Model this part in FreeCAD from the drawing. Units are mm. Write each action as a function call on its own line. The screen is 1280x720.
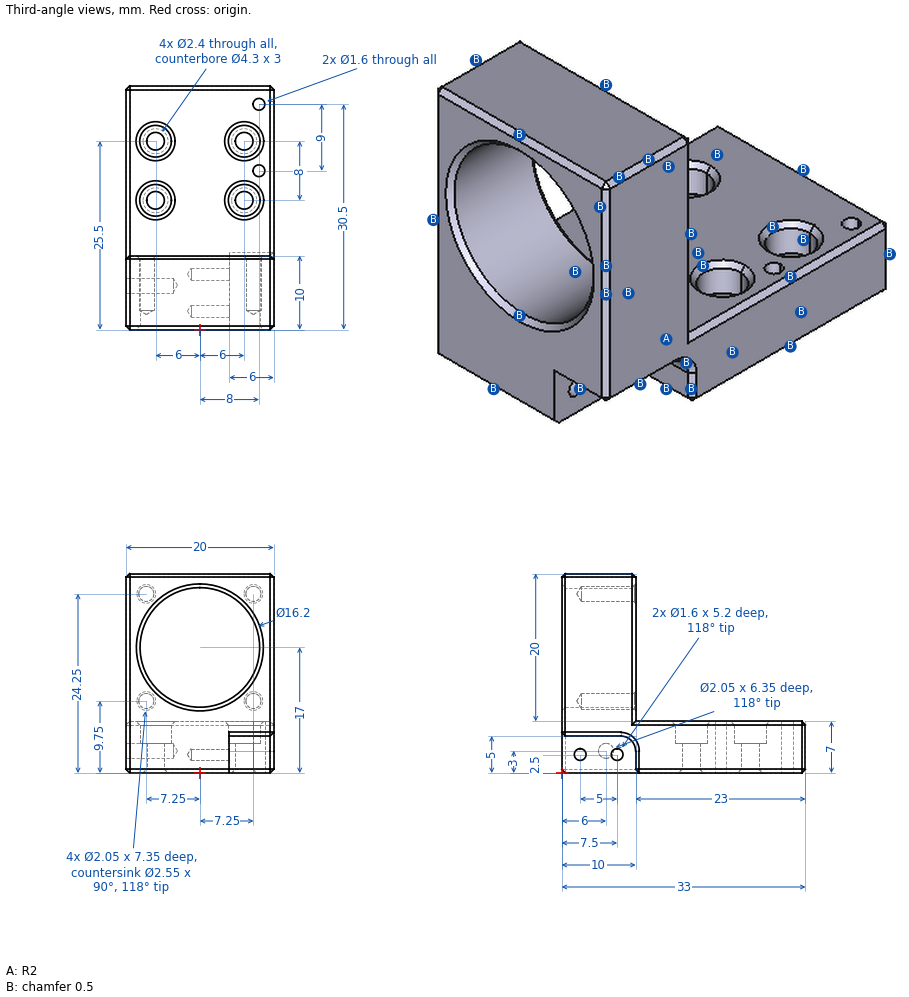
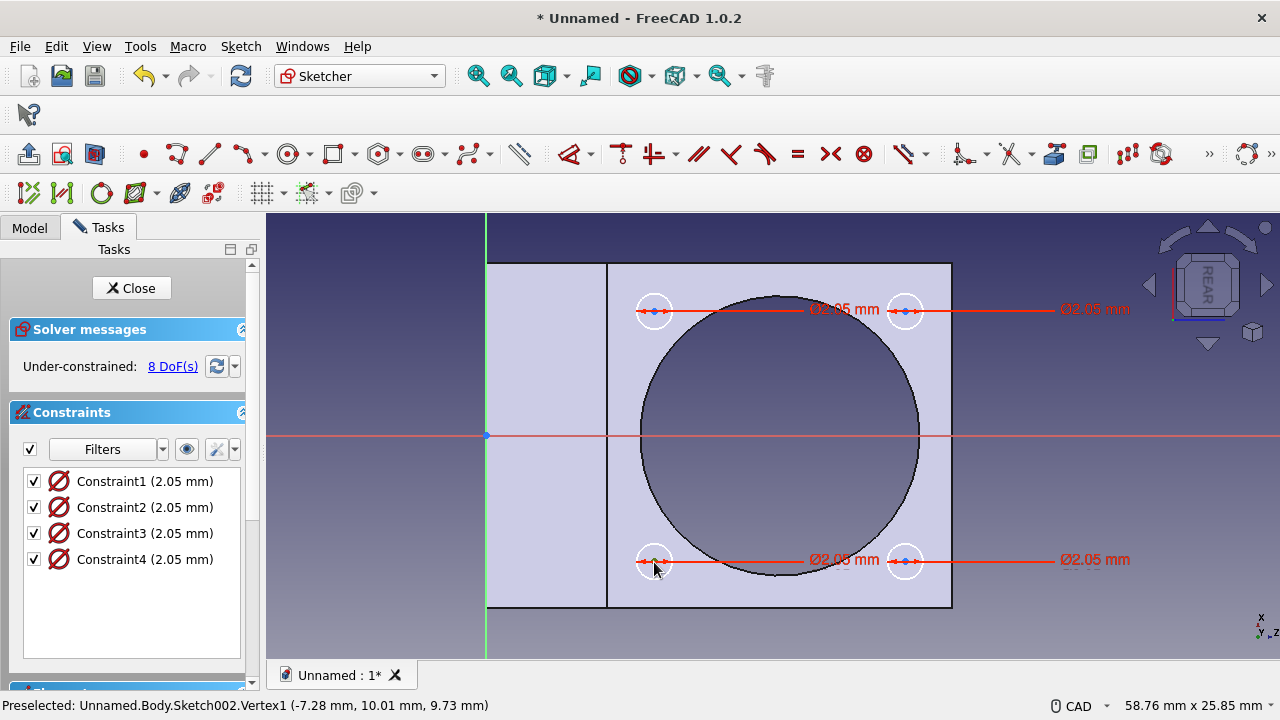
click(905, 562)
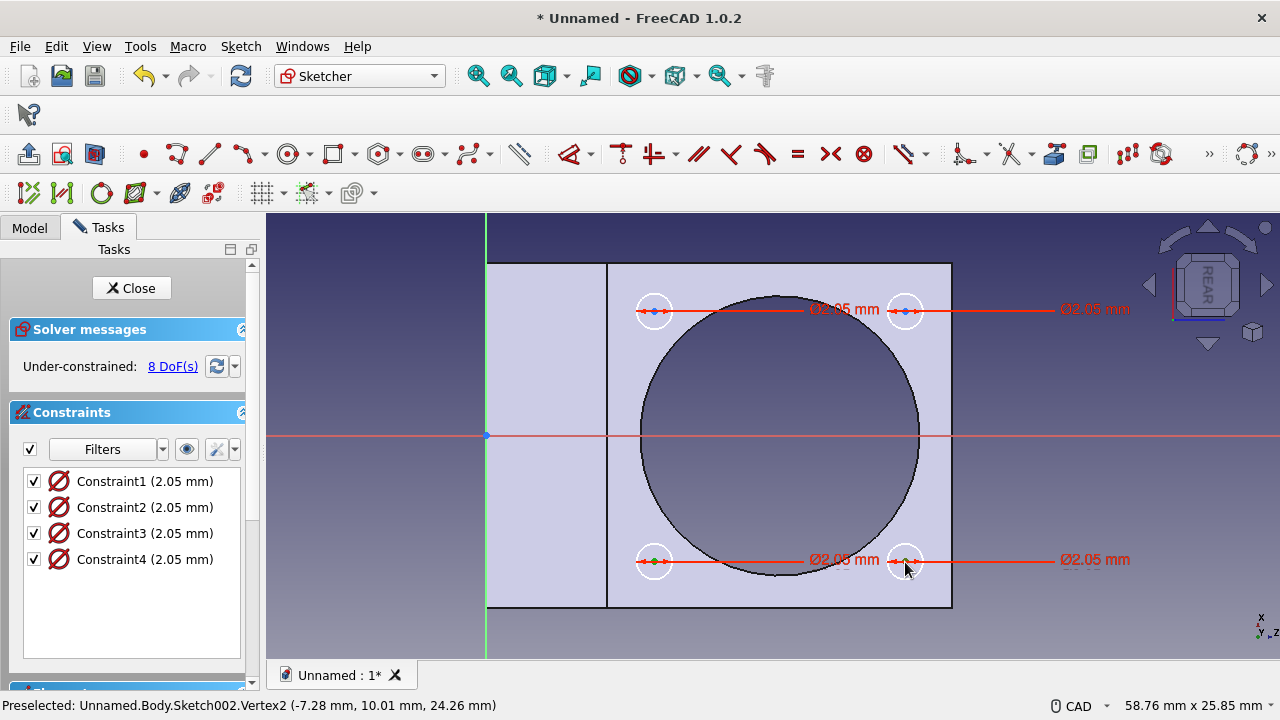
key(h)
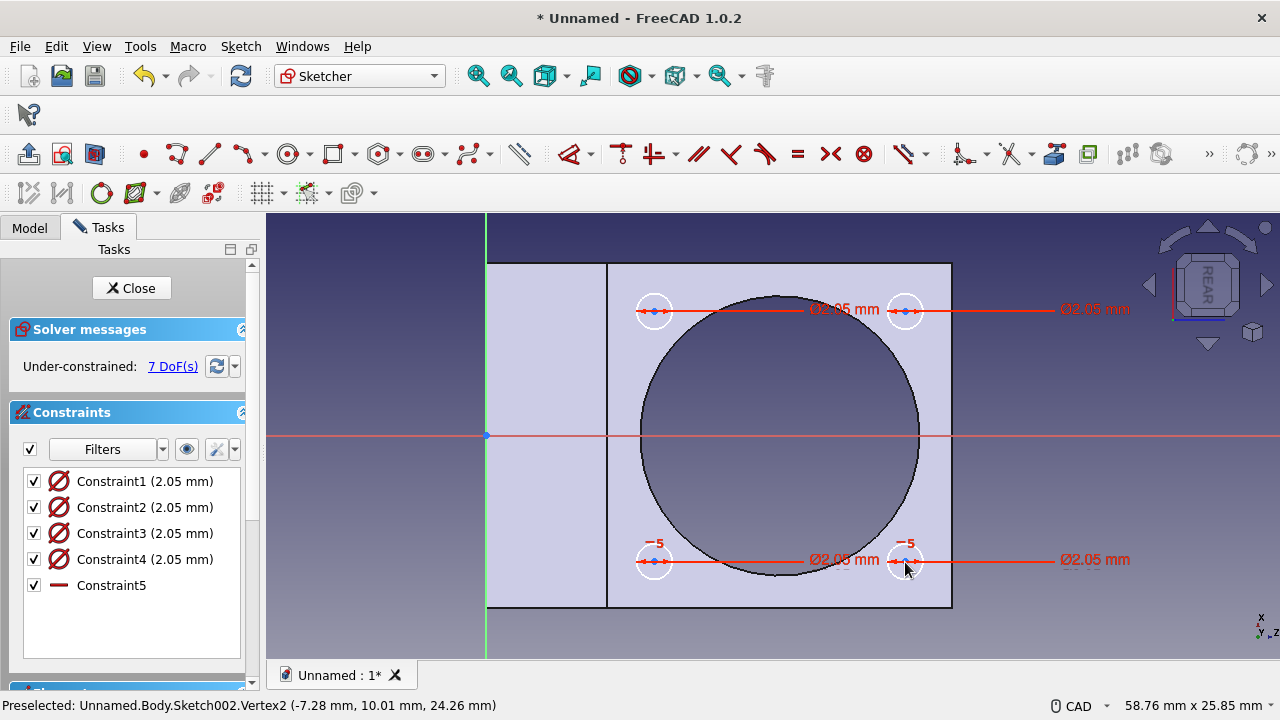
click(905, 562)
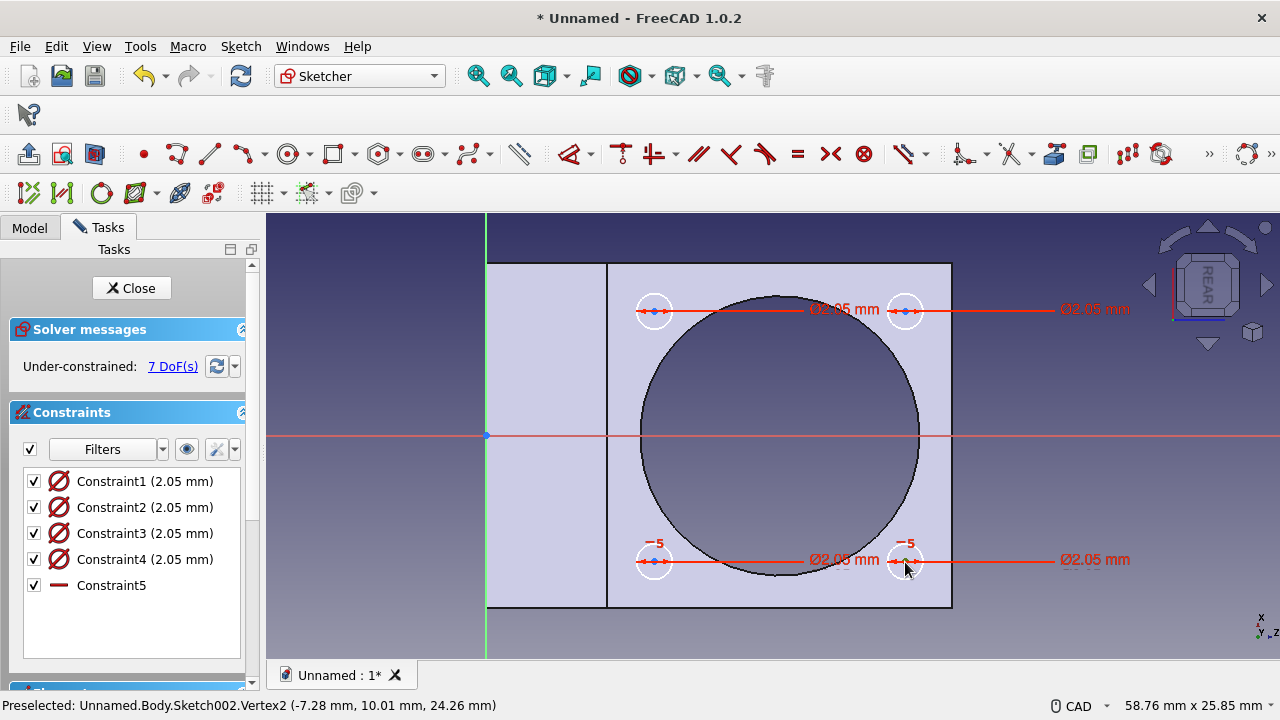
click(905, 311)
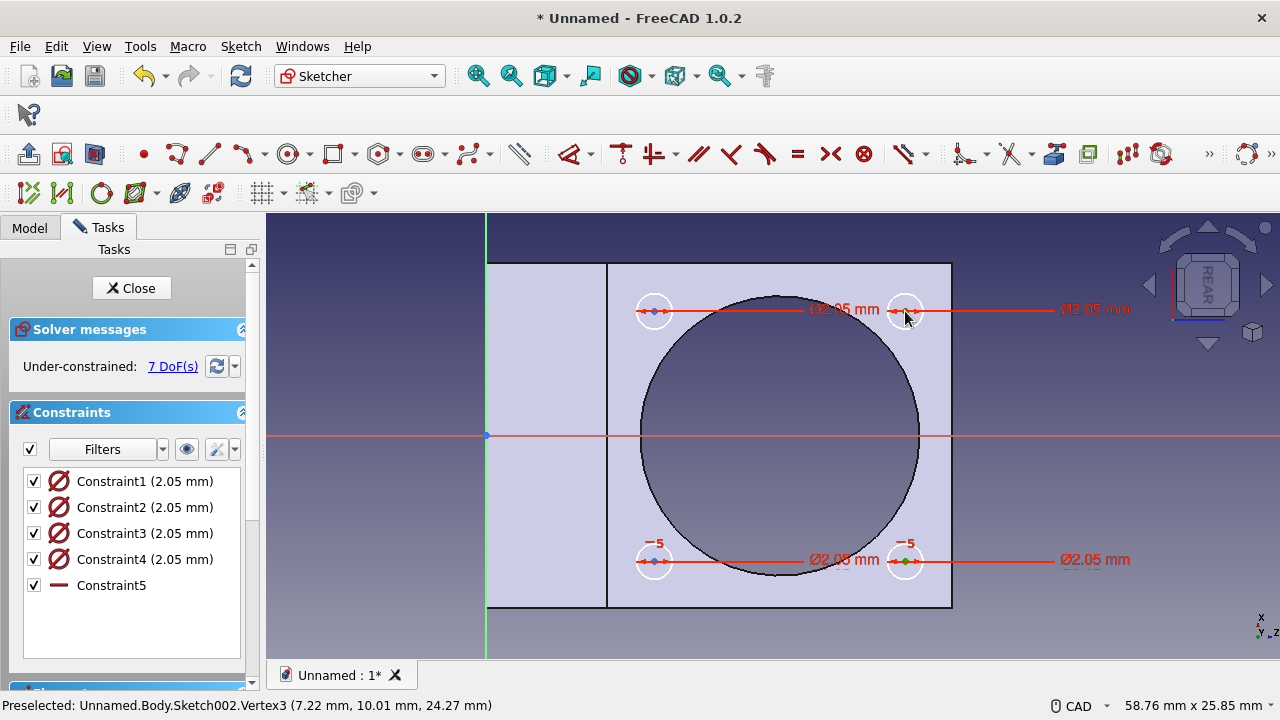
key(v)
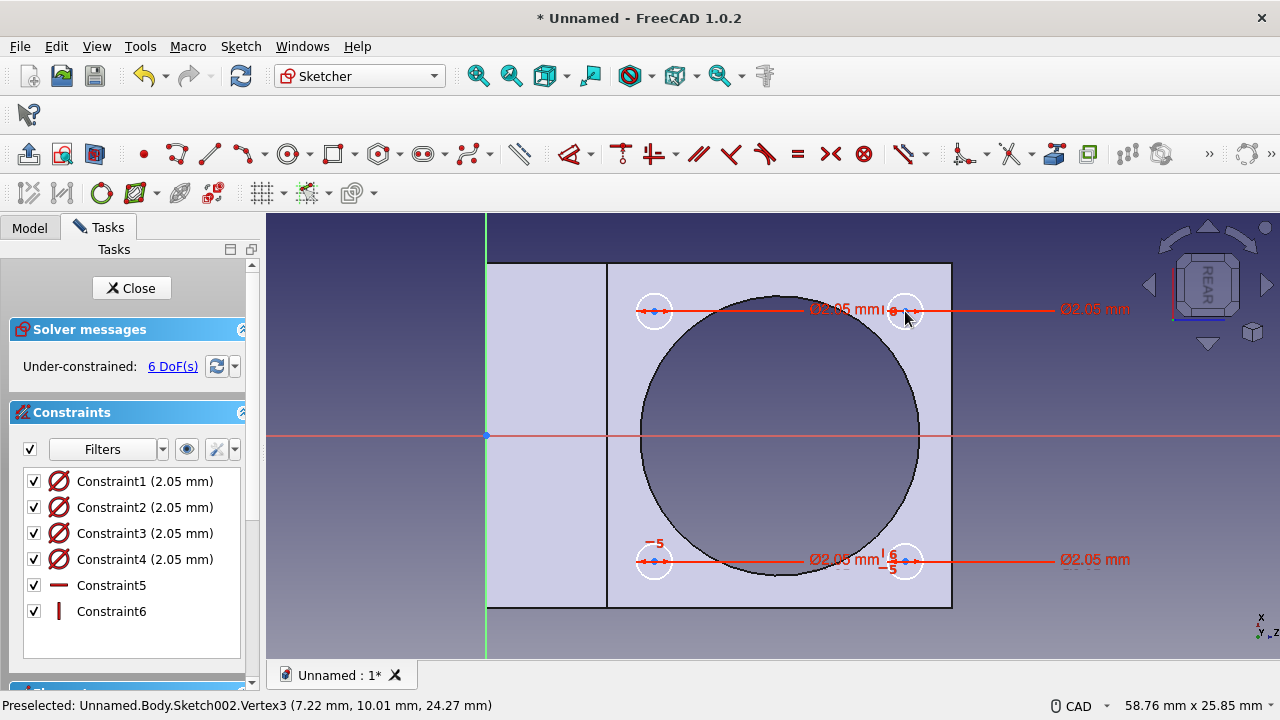
click(654, 562)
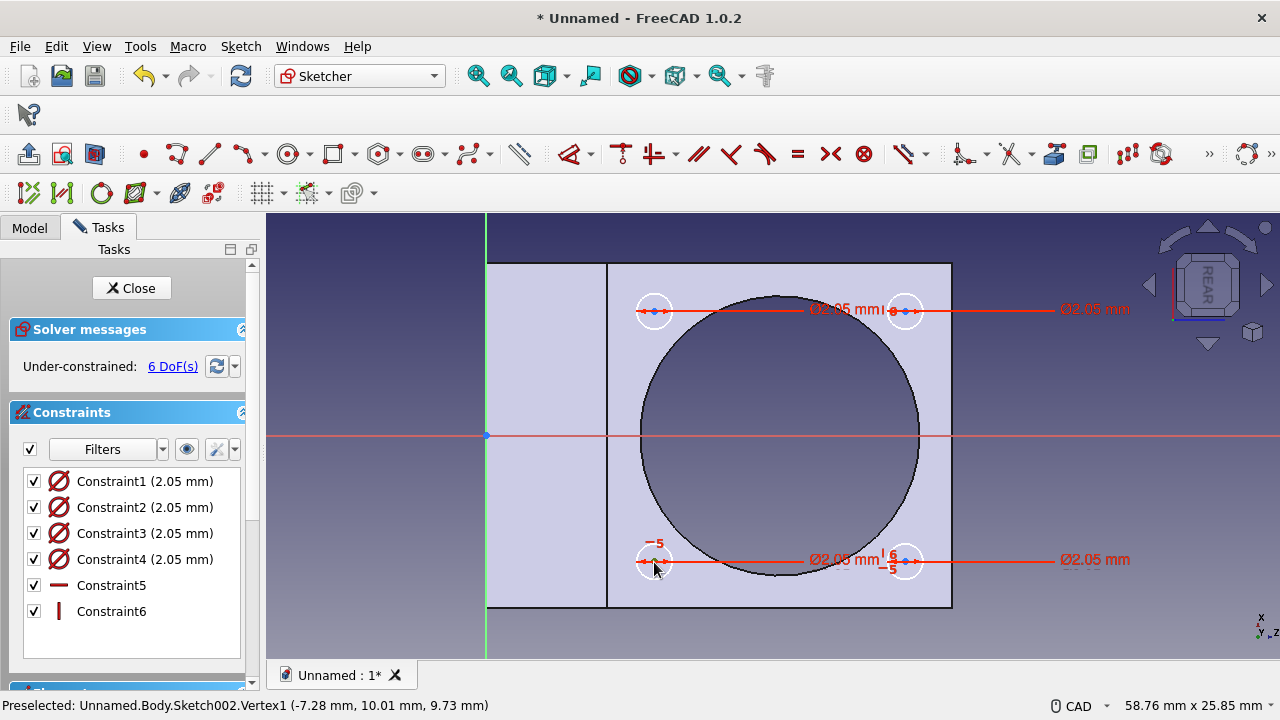
click(655, 311)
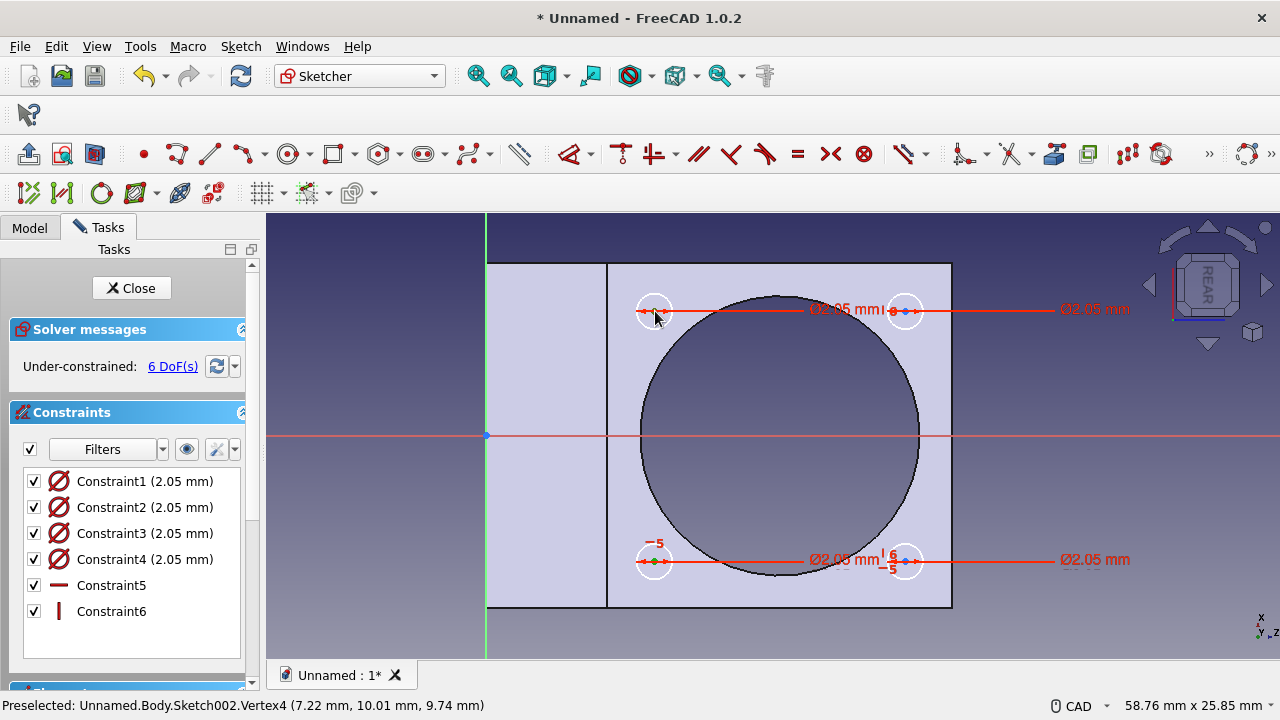
click(676, 154)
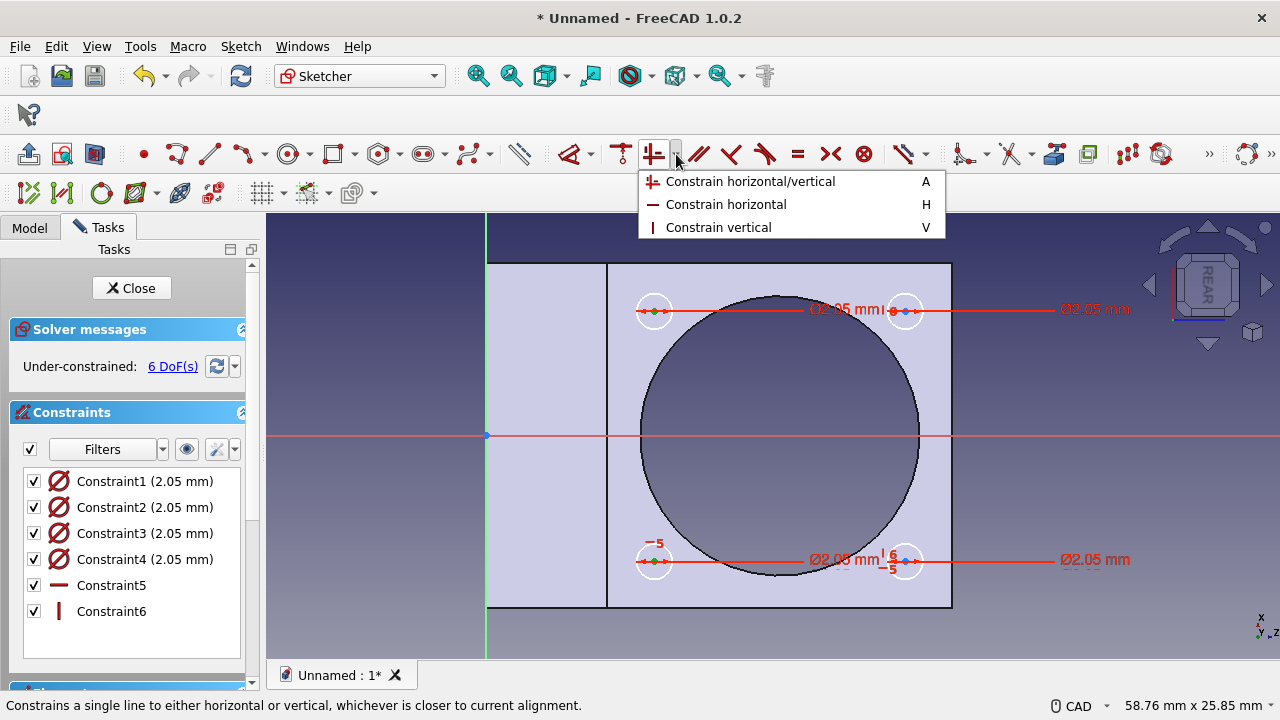
click(792, 228)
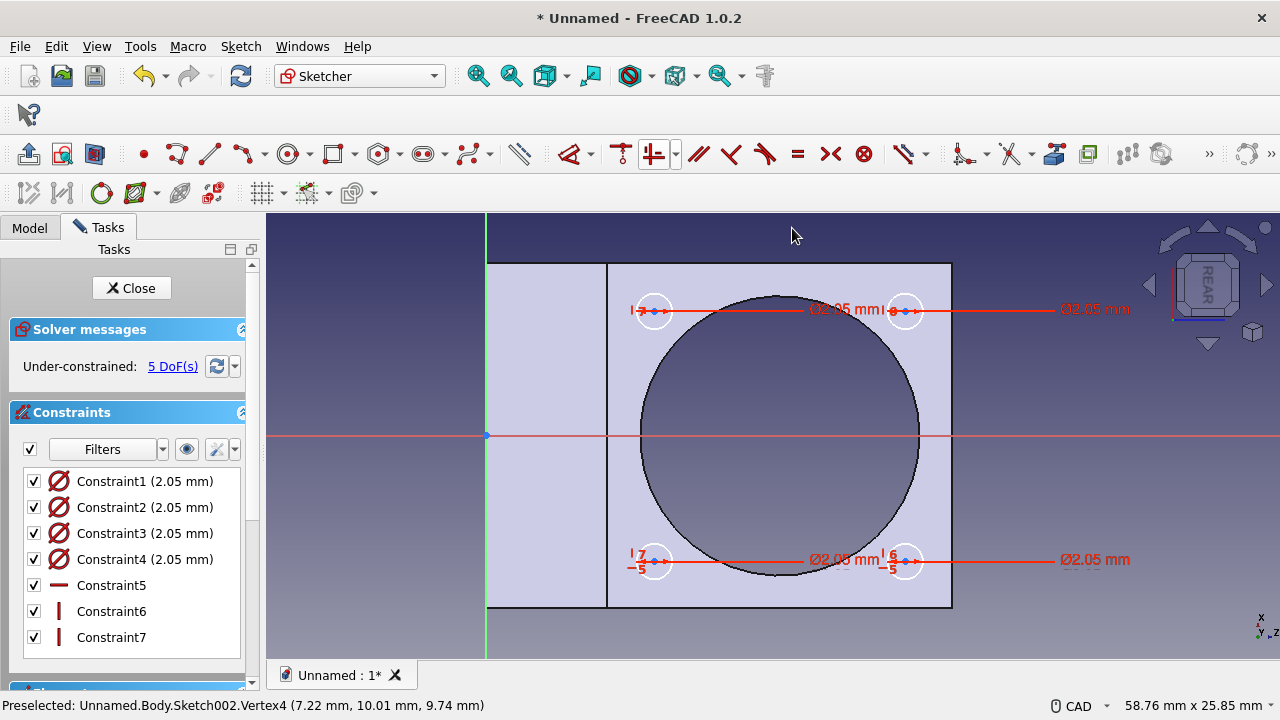
click(905, 311)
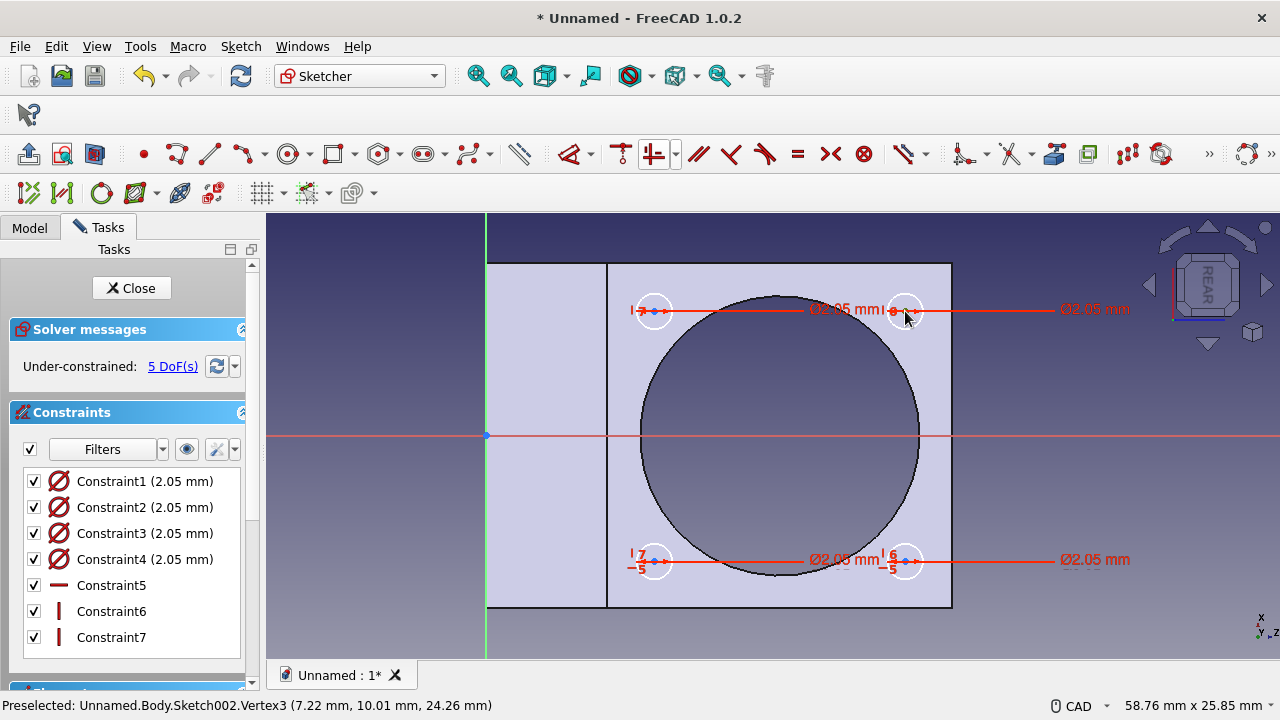
click(654, 311)